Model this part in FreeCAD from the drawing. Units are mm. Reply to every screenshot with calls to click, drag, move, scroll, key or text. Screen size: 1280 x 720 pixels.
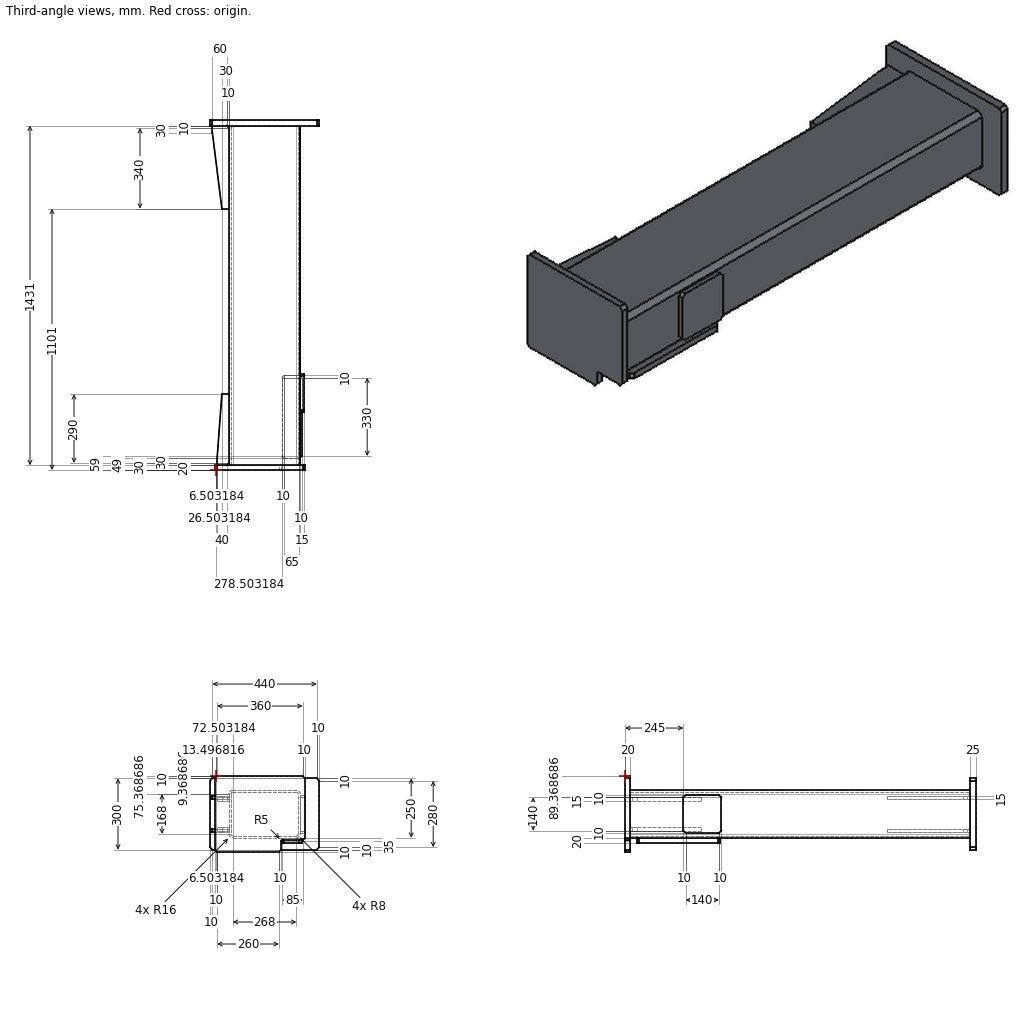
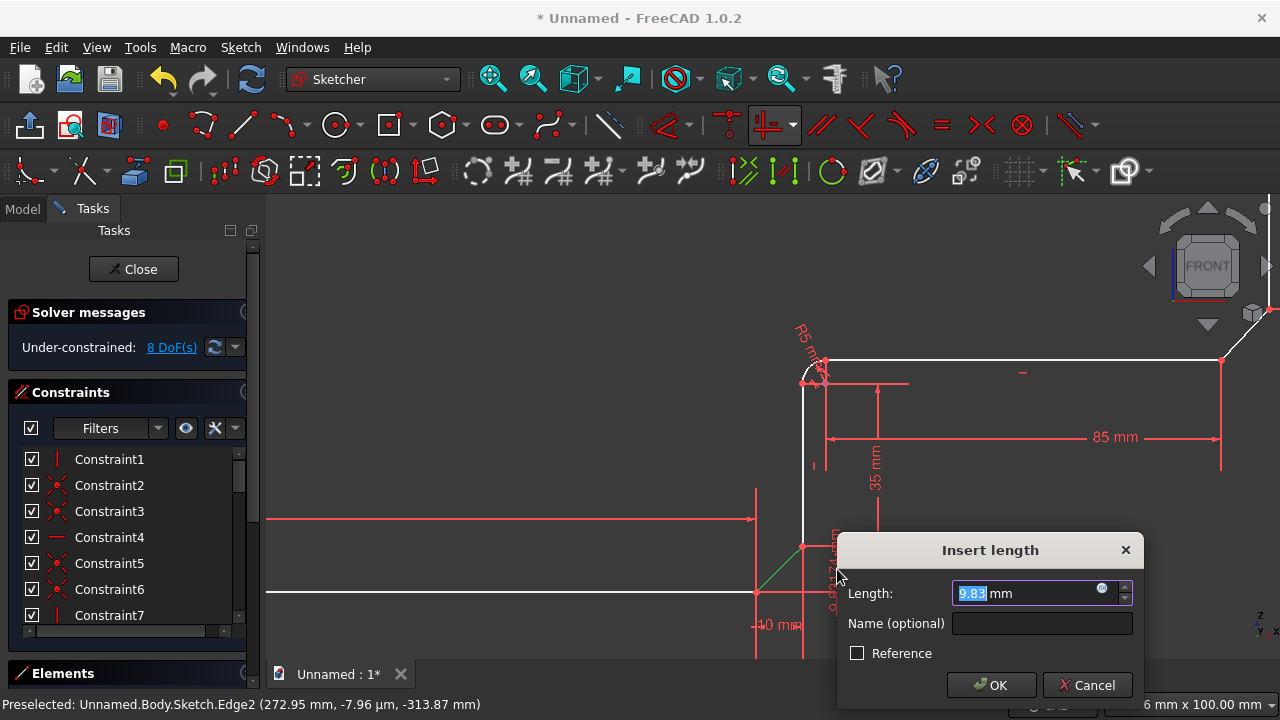
text(10)
key(Return)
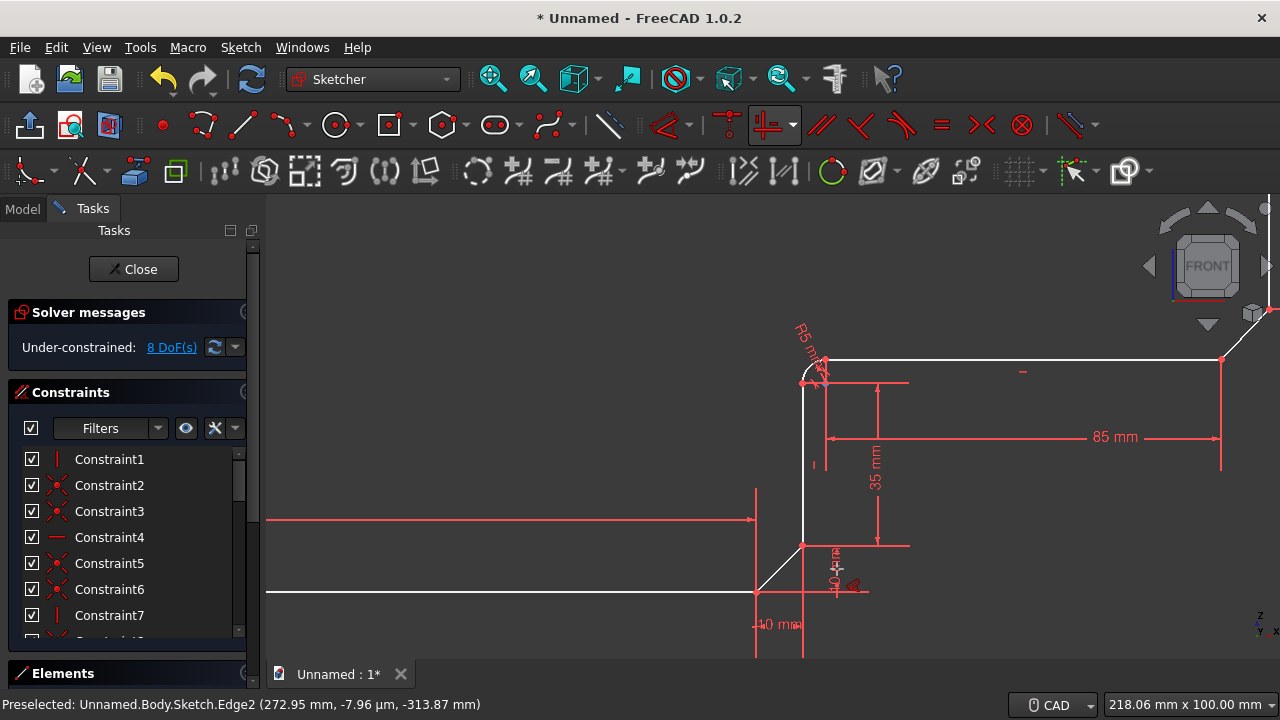
scroll(785, 574, down, 8)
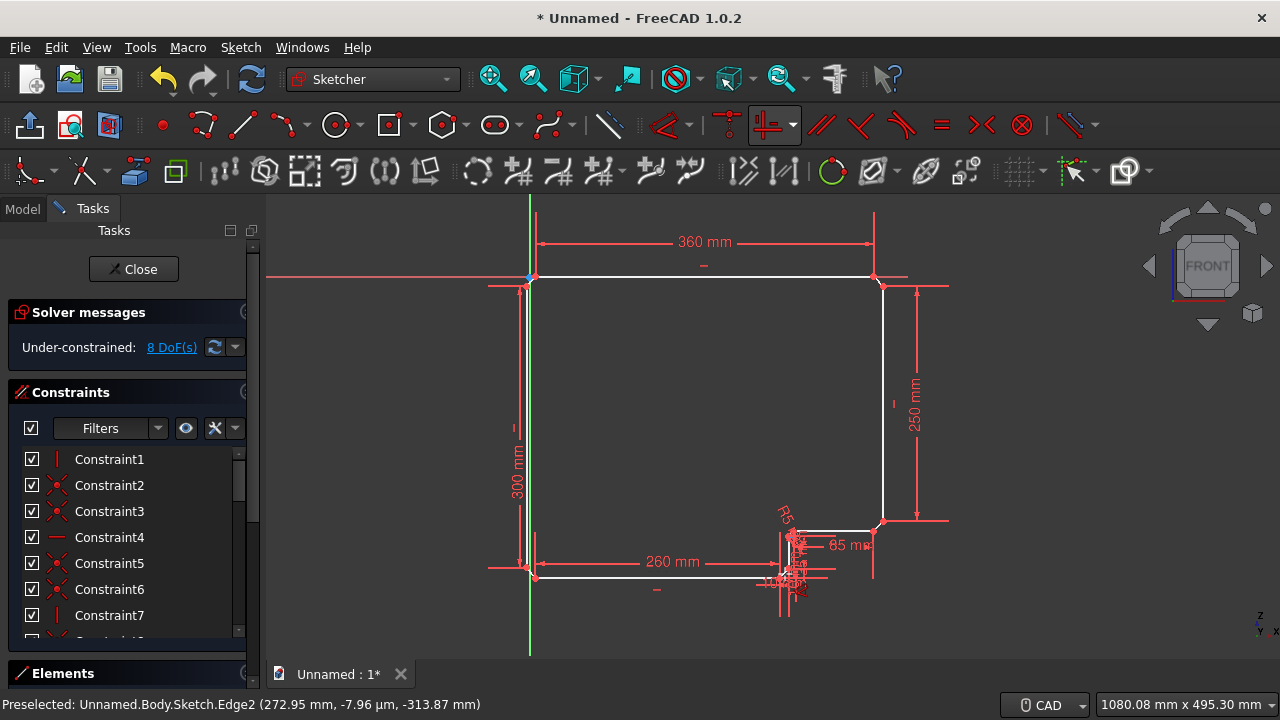
scroll(533, 575, up, 8)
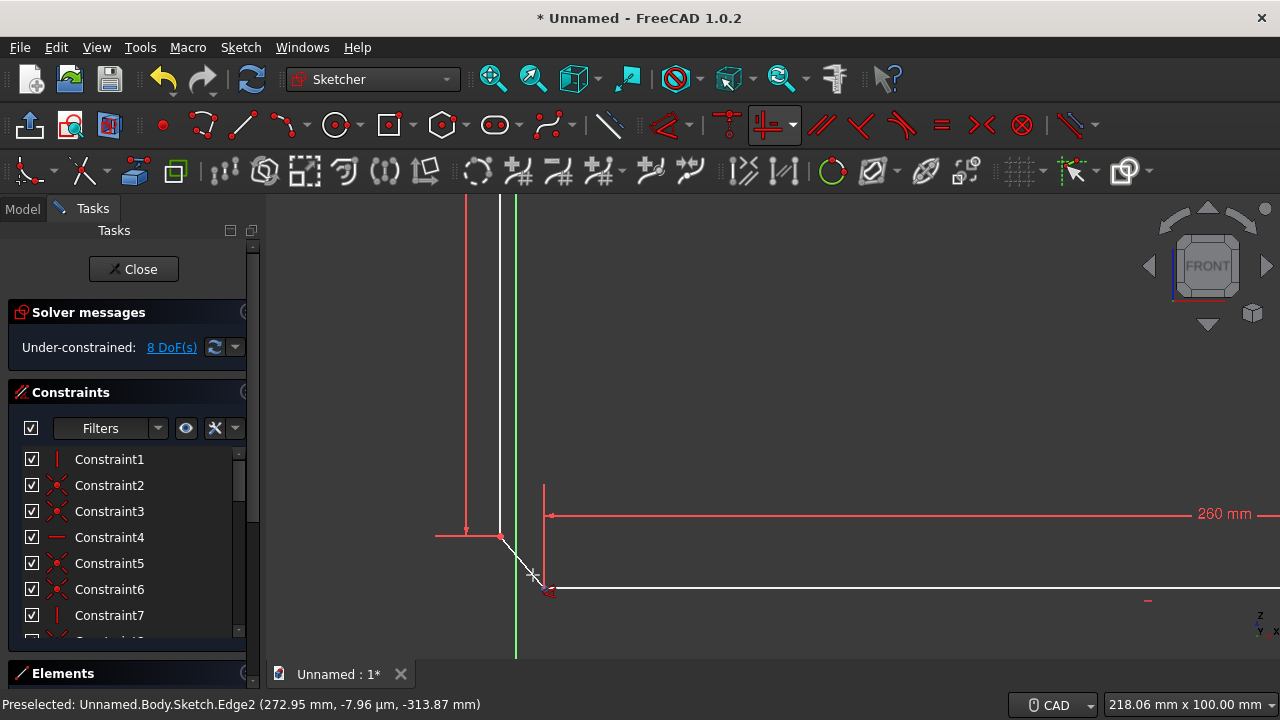
click(531, 573)
click(532, 622)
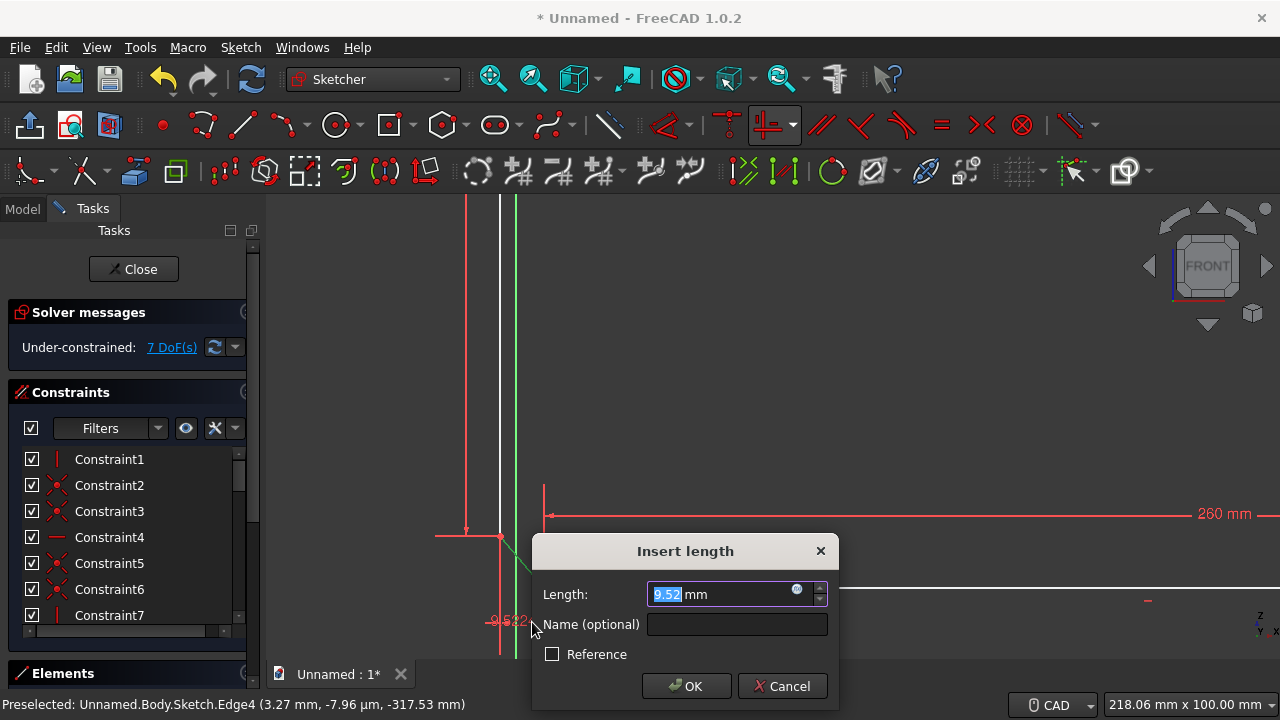
text(10)
key(Return)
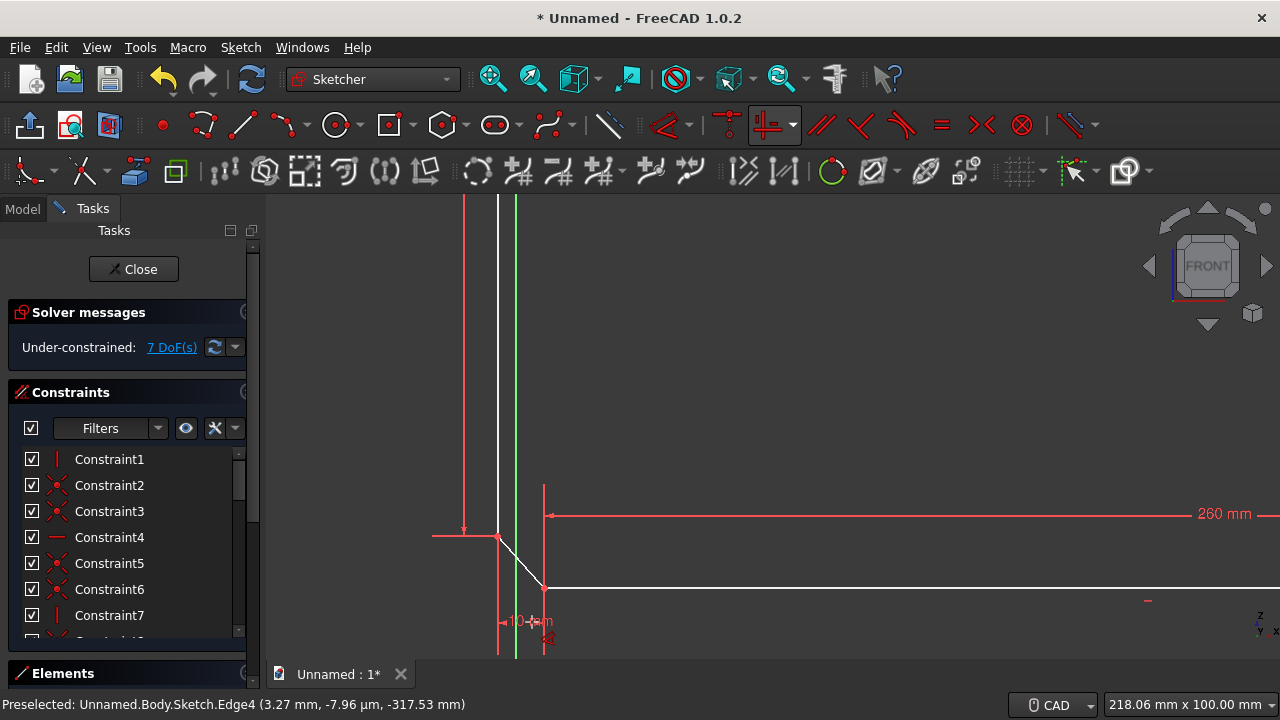
click(530, 573)
click(464, 562)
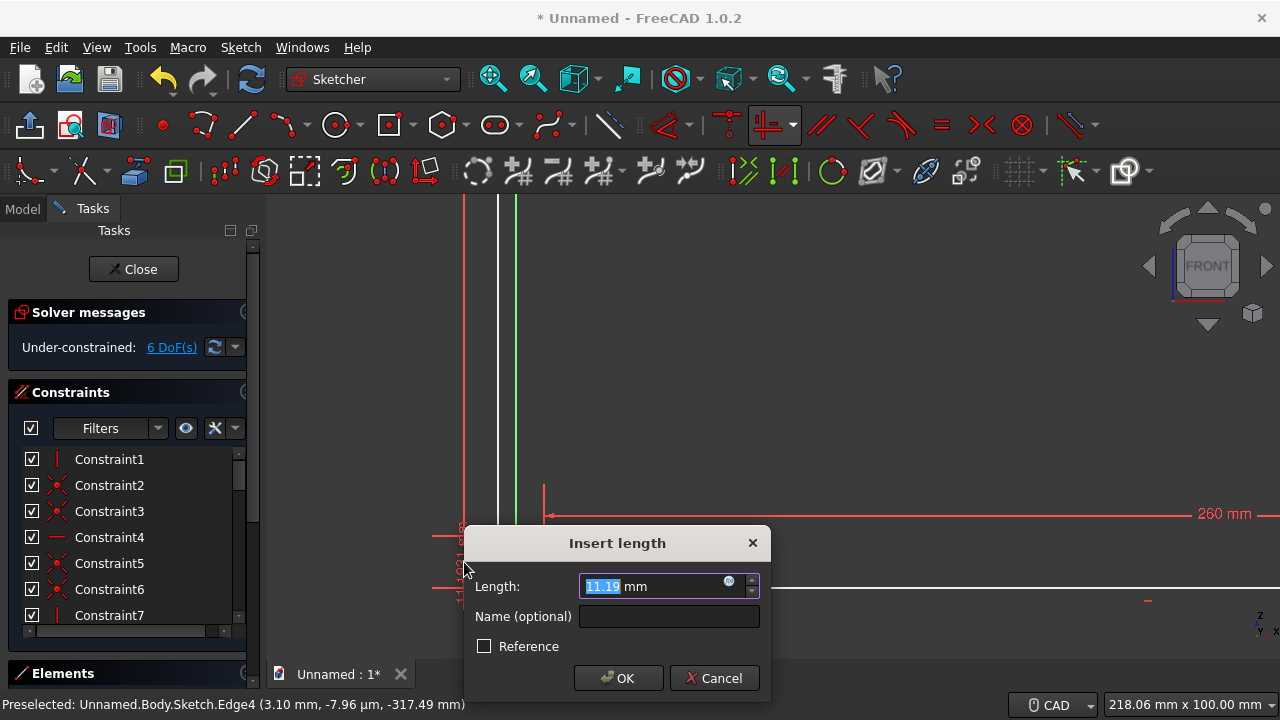
text(10)
key(Return)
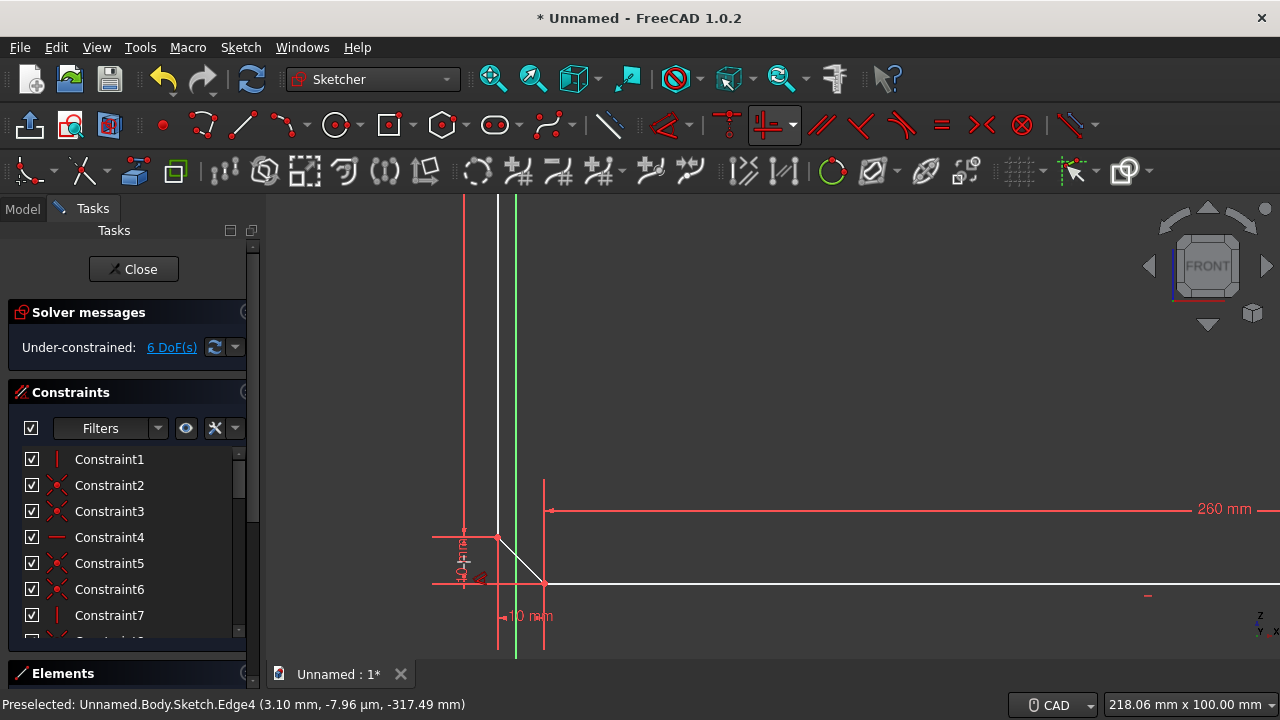
scroll(533, 575, down, 8)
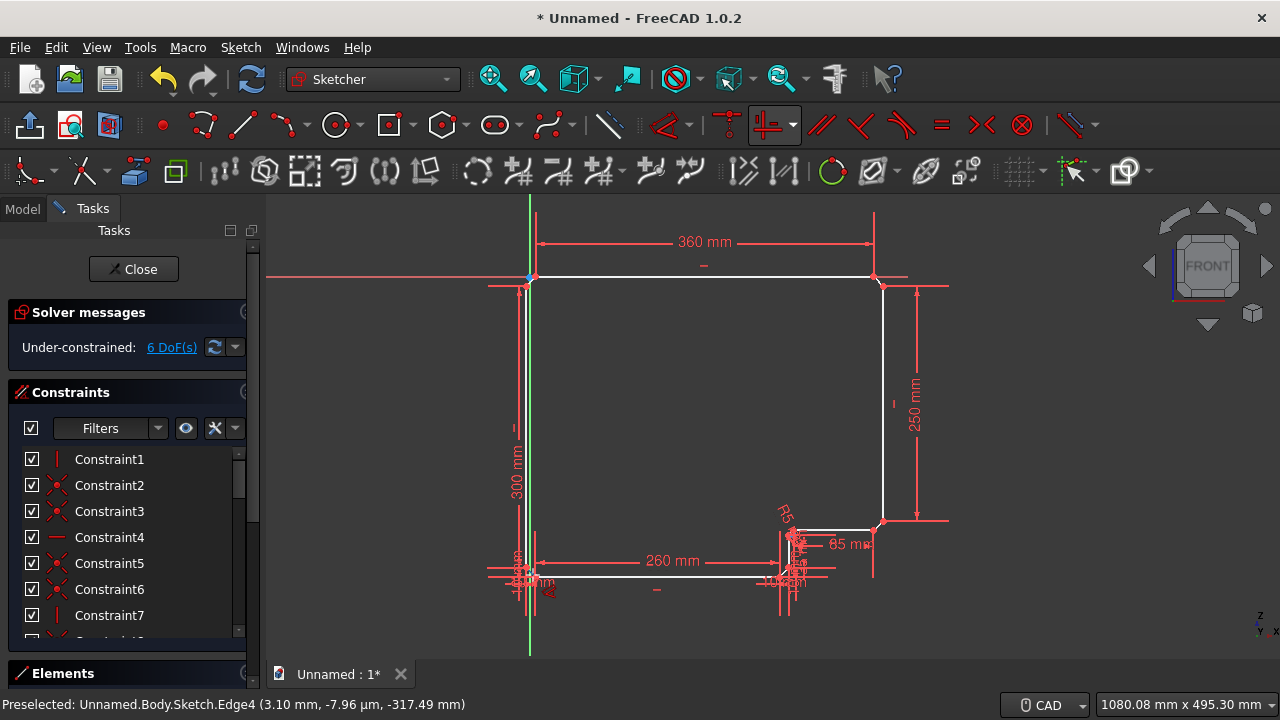
scroll(529, 283, up, 8)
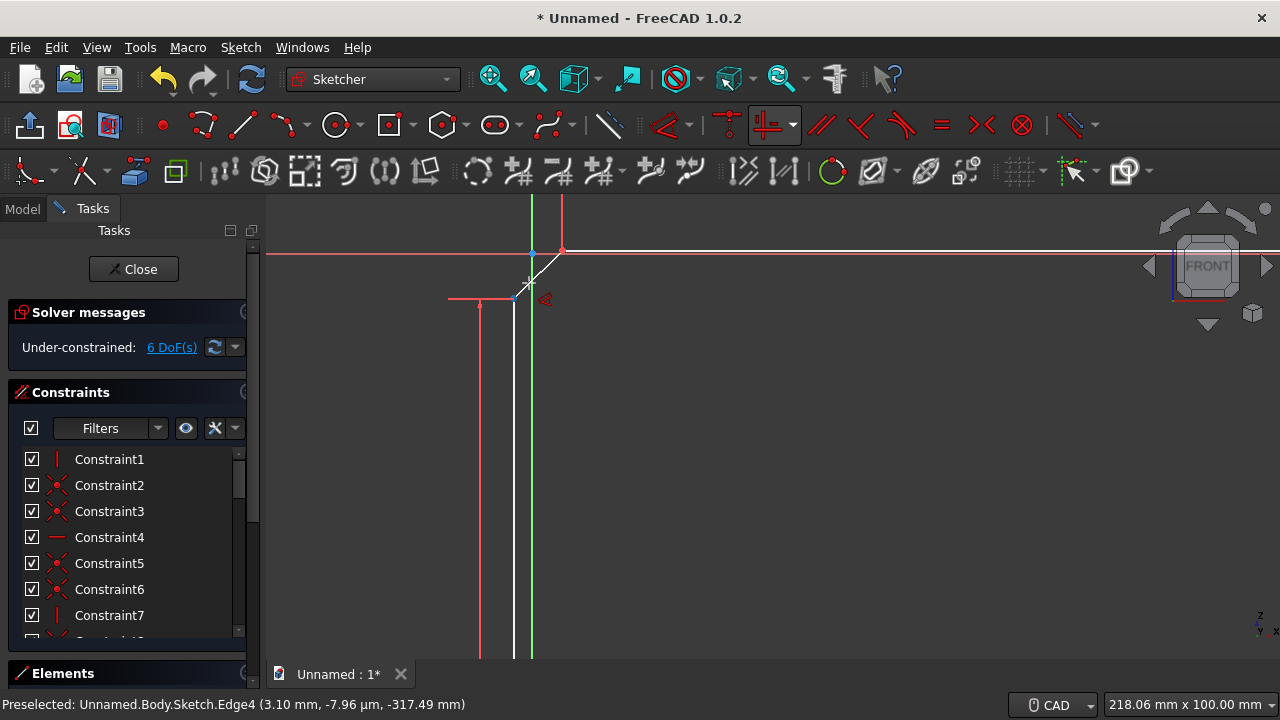
click(528, 284)
click(549, 333)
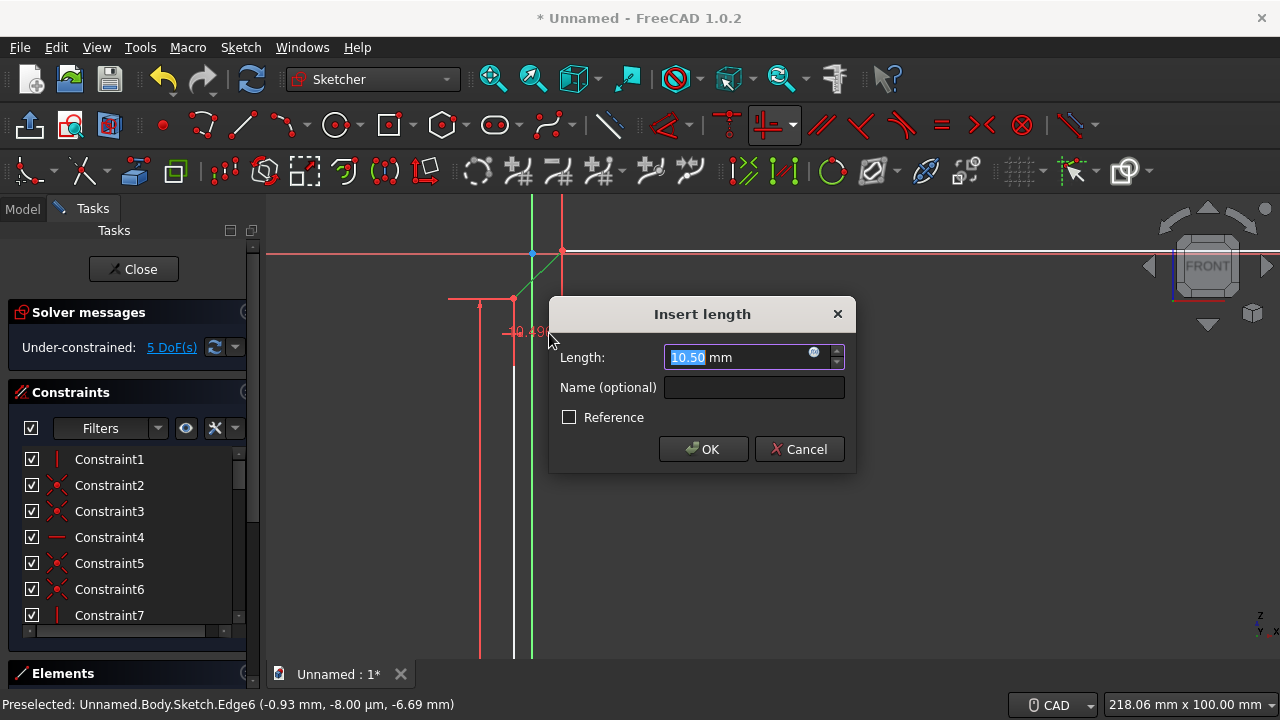
text(10)
key(Return)